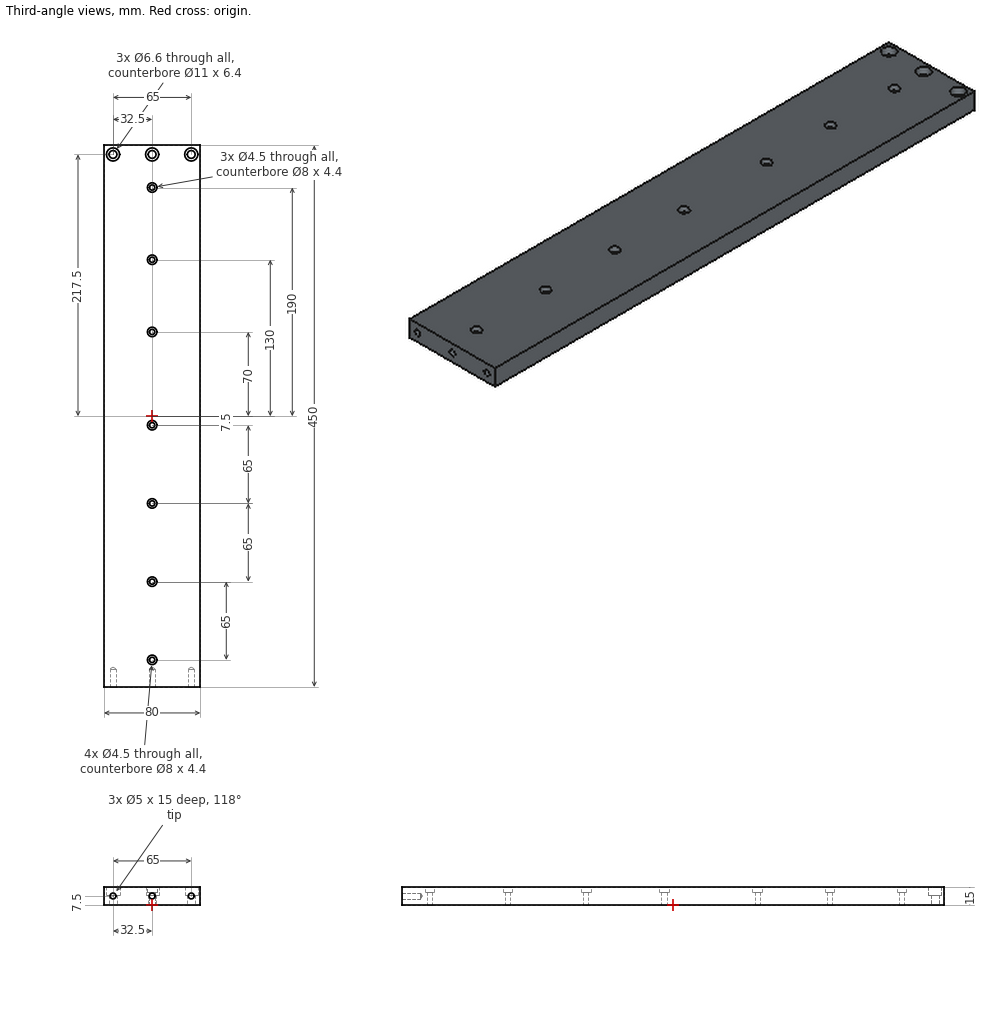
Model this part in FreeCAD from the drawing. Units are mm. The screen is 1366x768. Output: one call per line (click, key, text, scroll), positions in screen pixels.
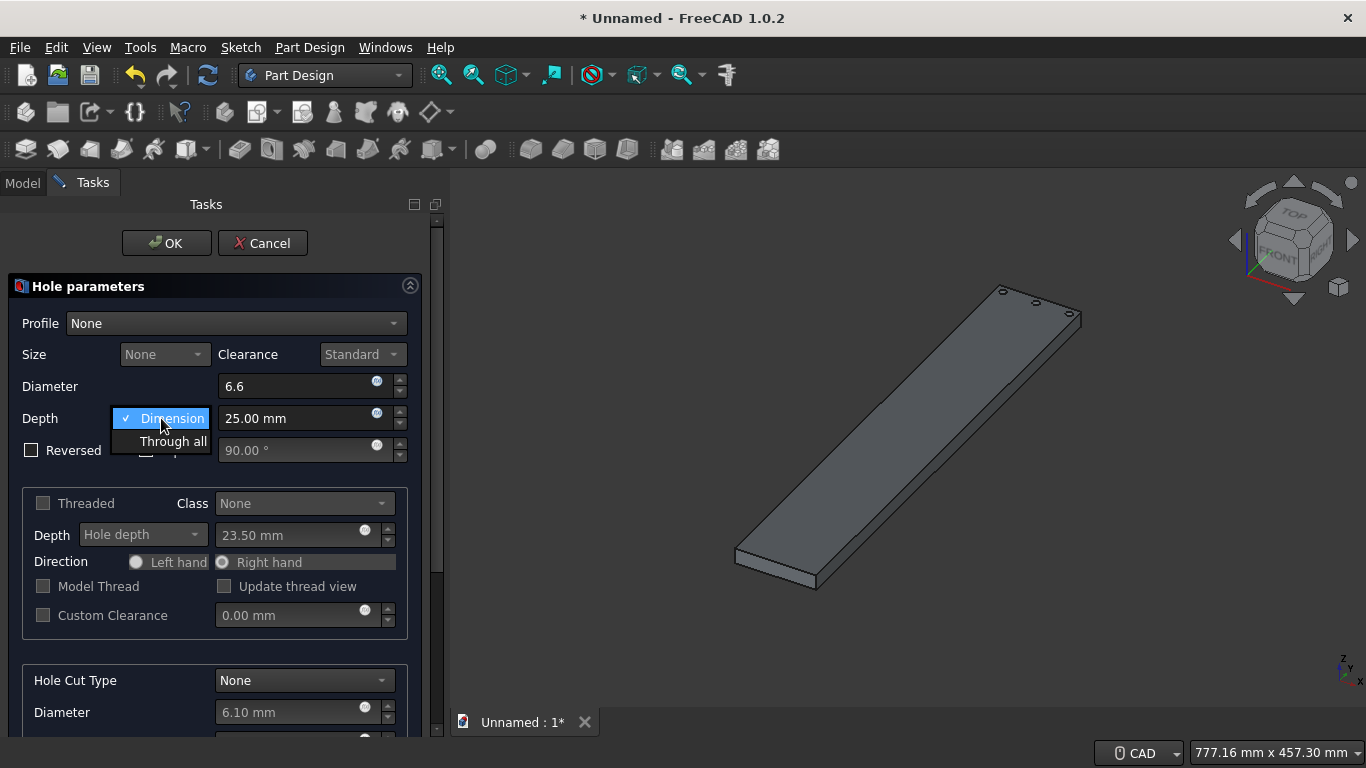
click(160, 442)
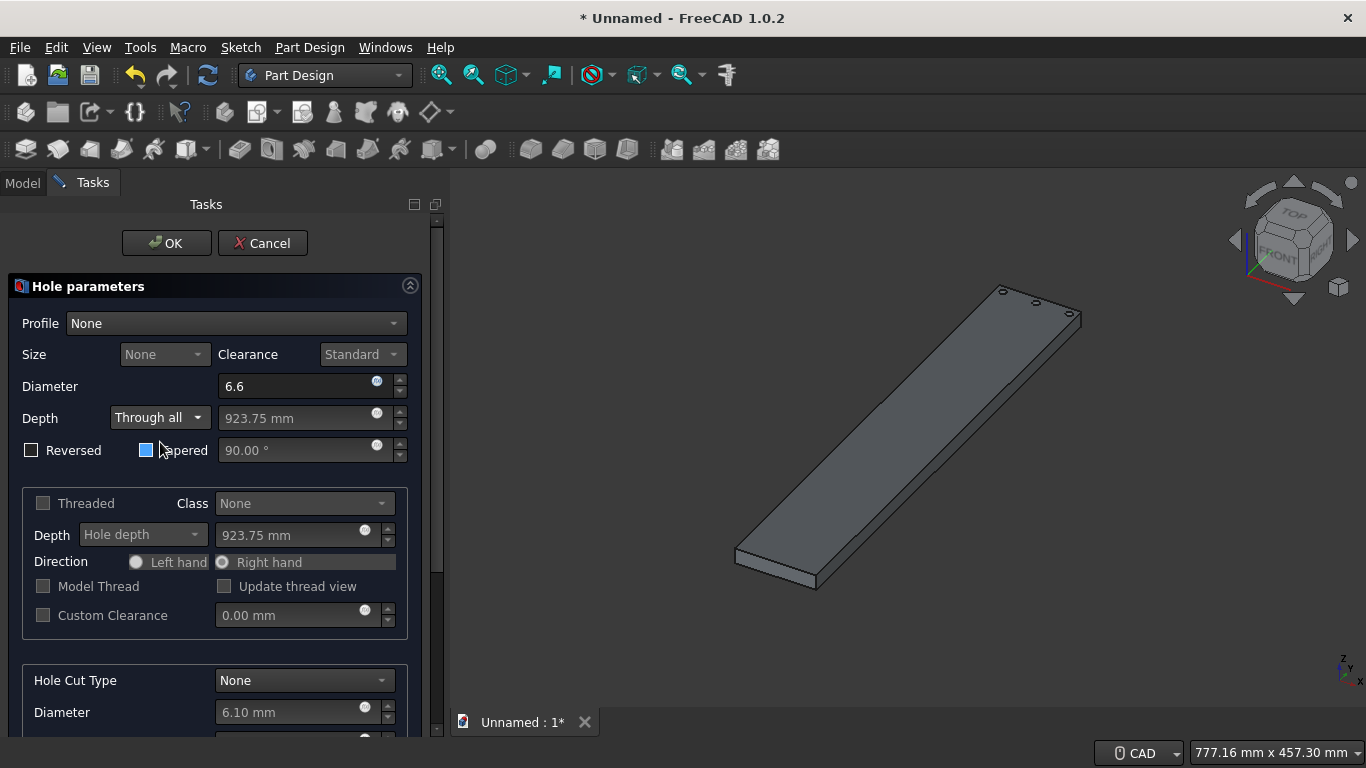
click(306, 680)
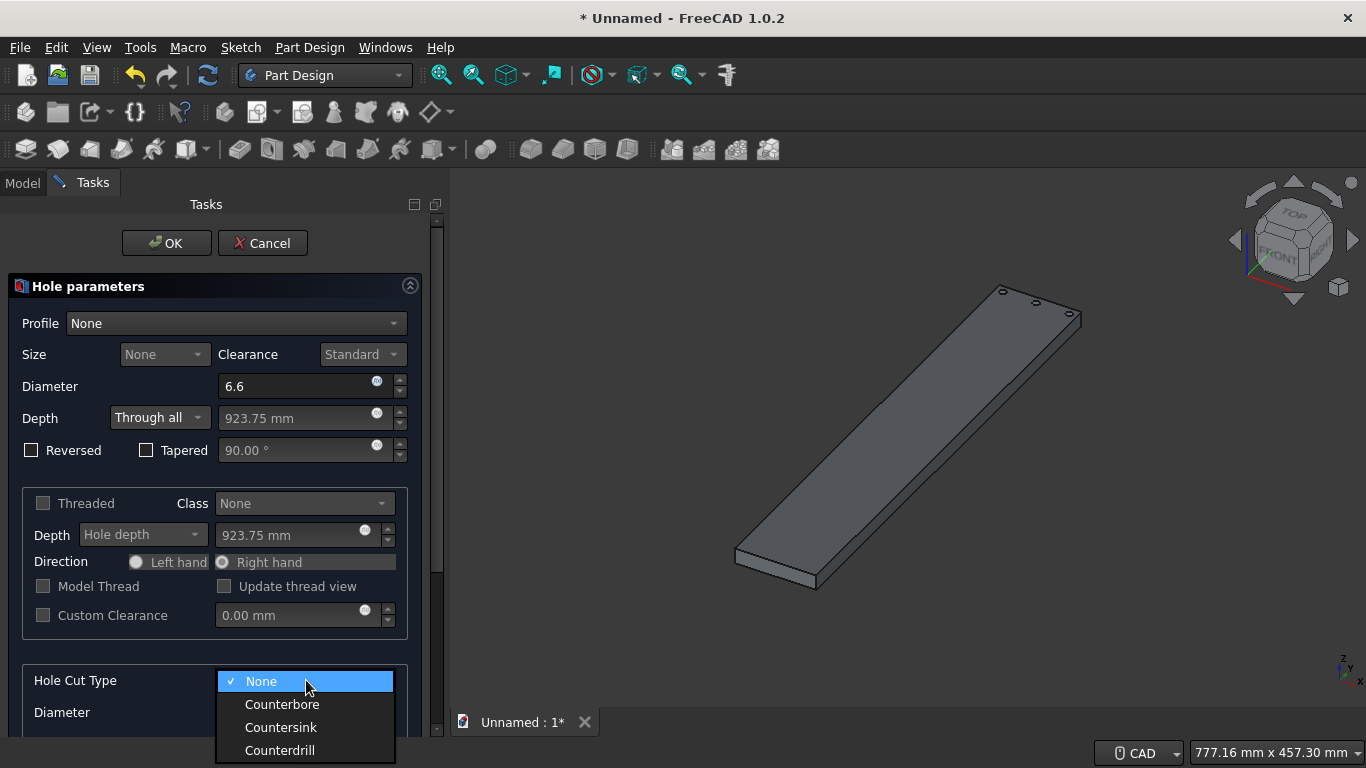
click(304, 704)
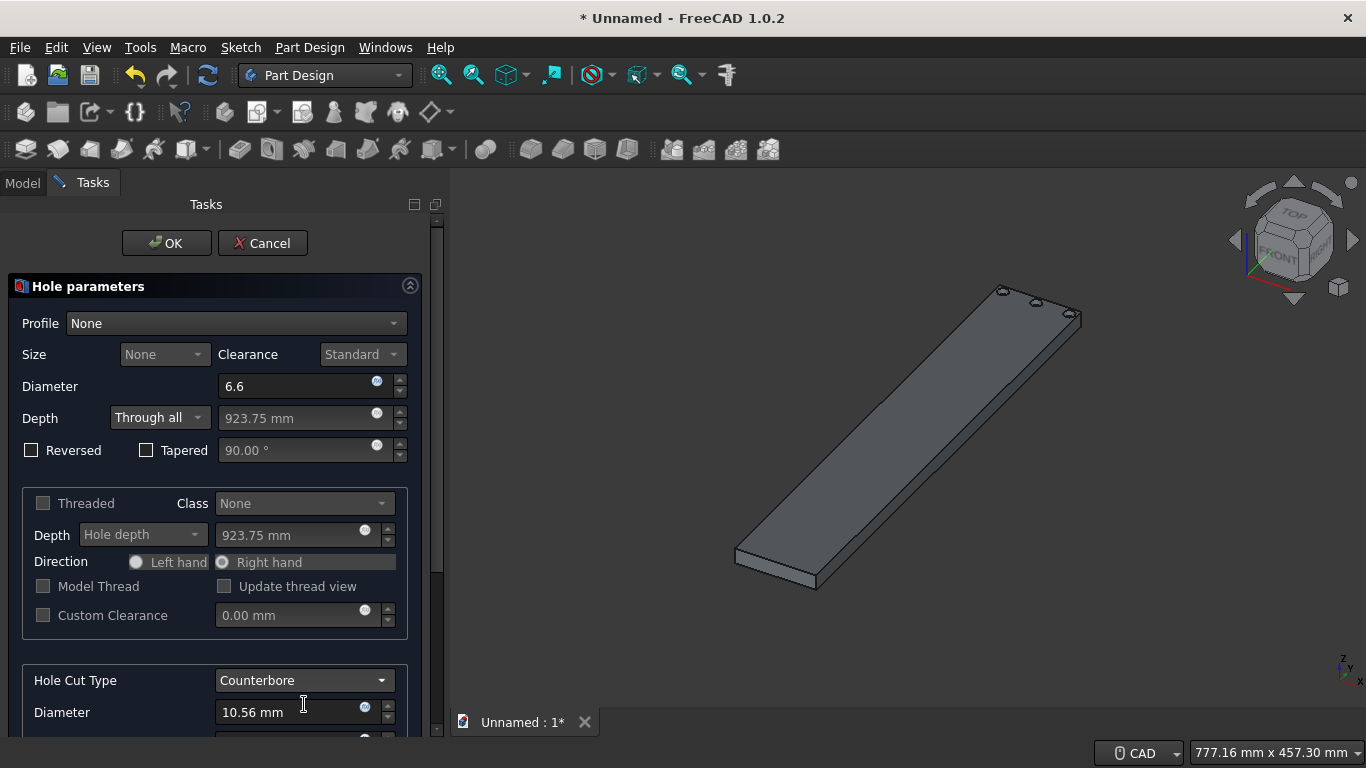
triple_click(298, 712)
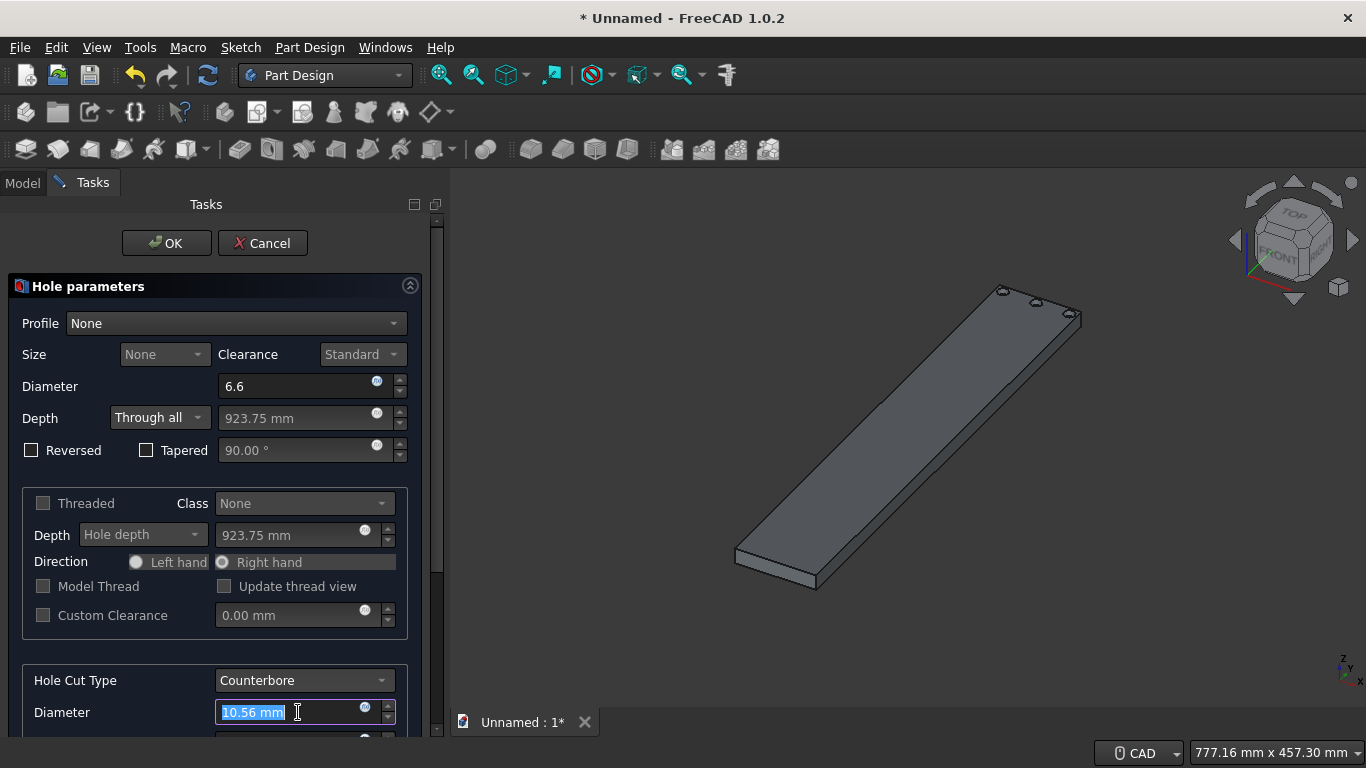
text(11)
key(Tab)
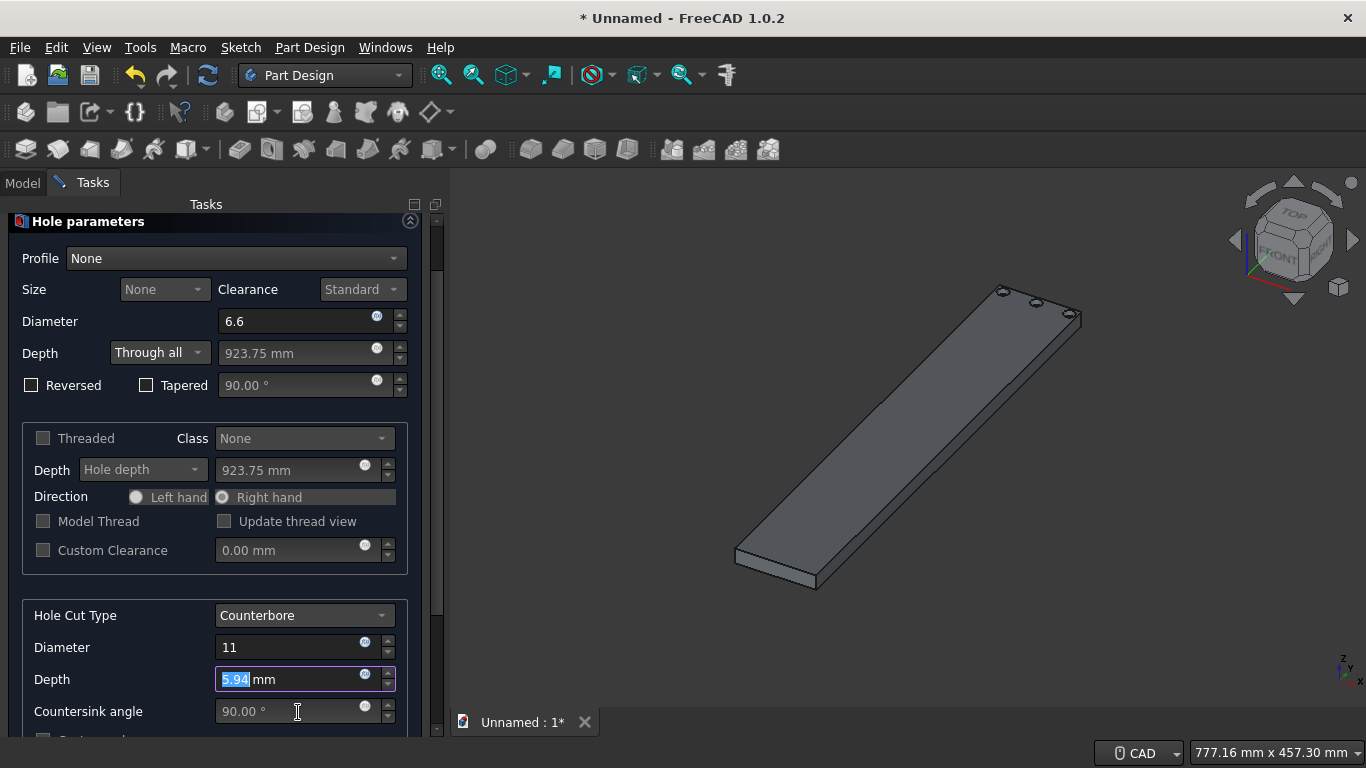
text(6.4)
key(Tab)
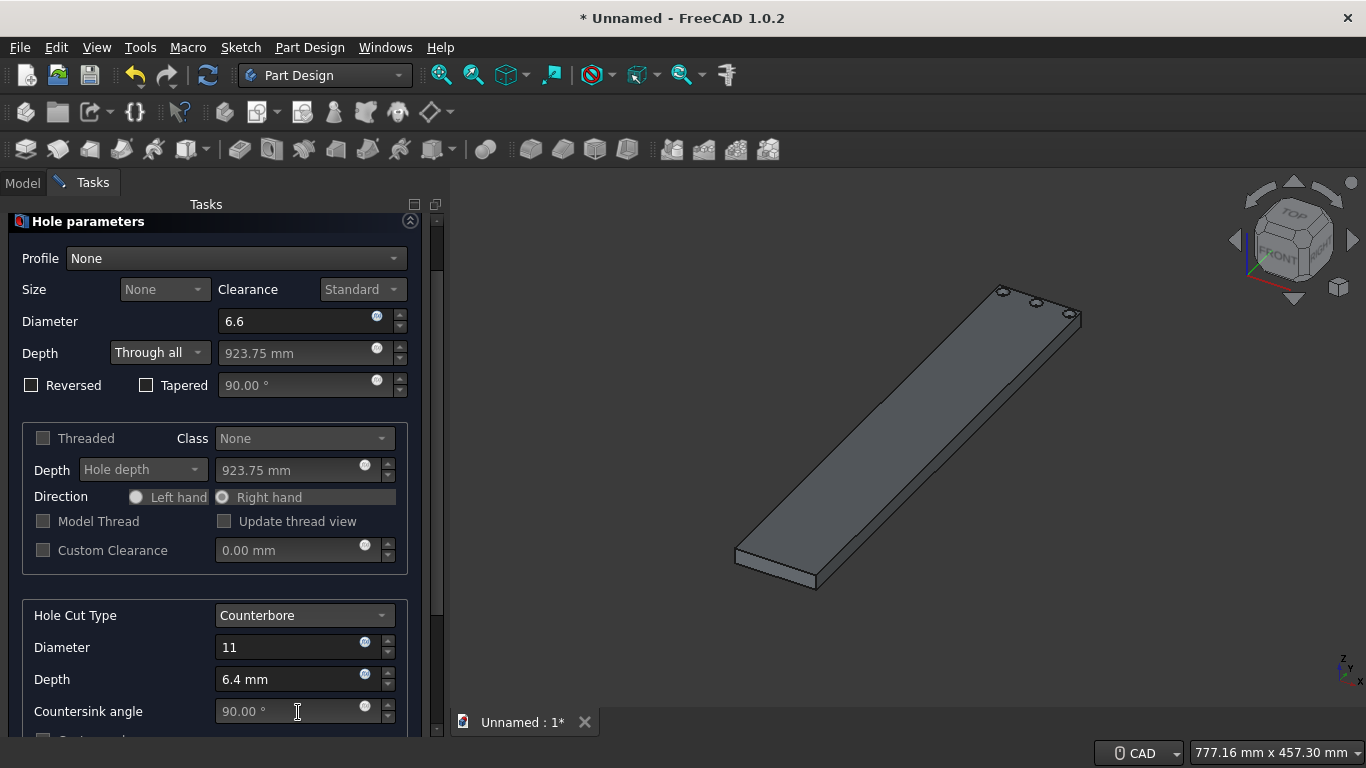
scroll(437, 475, up, 2)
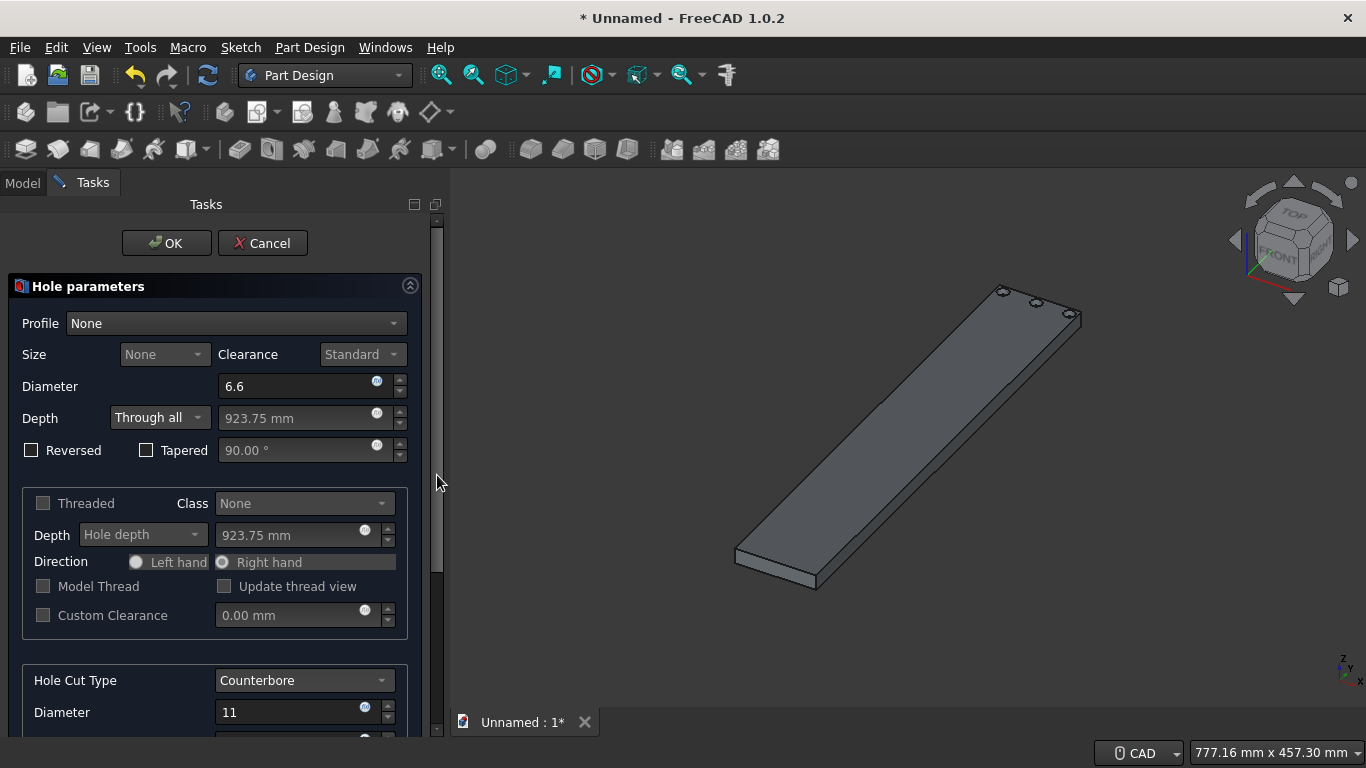
click(167, 243)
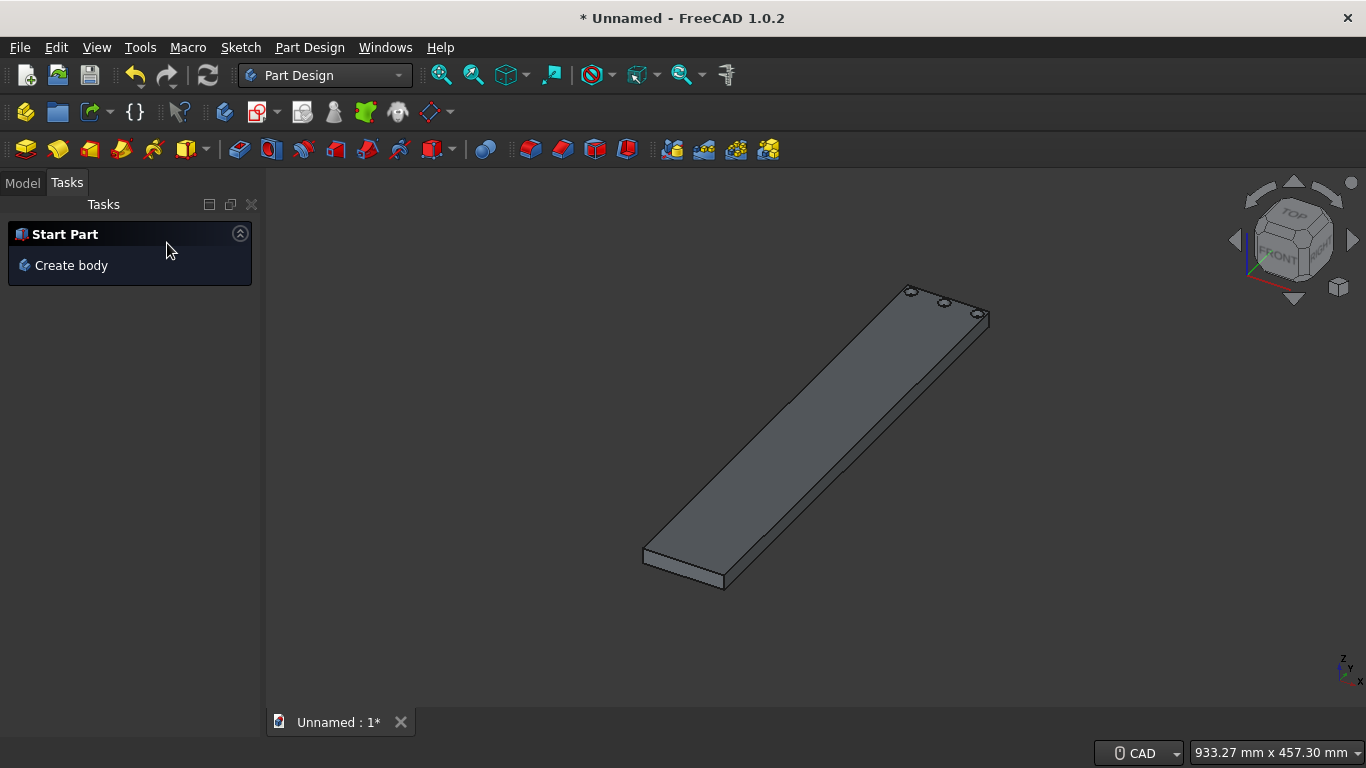
click(892, 354)